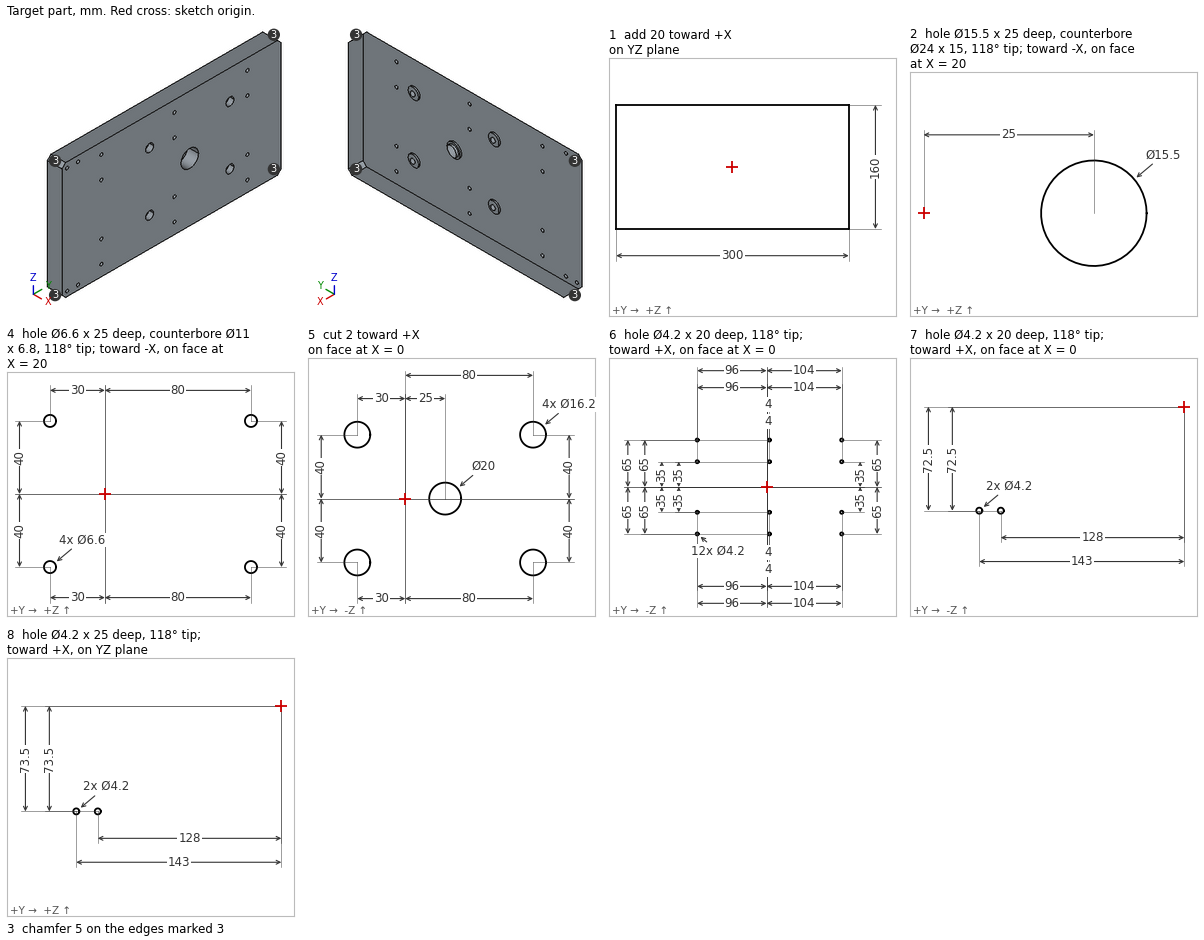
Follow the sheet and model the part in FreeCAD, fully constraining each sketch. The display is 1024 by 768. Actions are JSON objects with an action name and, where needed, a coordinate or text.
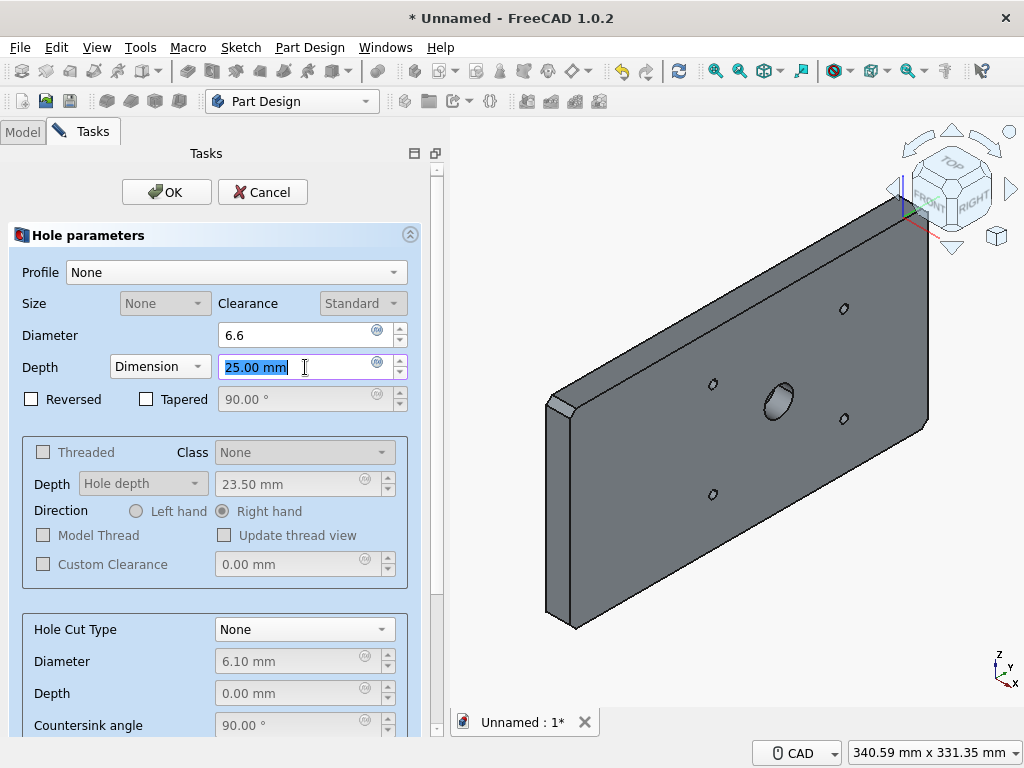
{"action": "type", "text": "25"}
{"action": "key", "text": "Tab"}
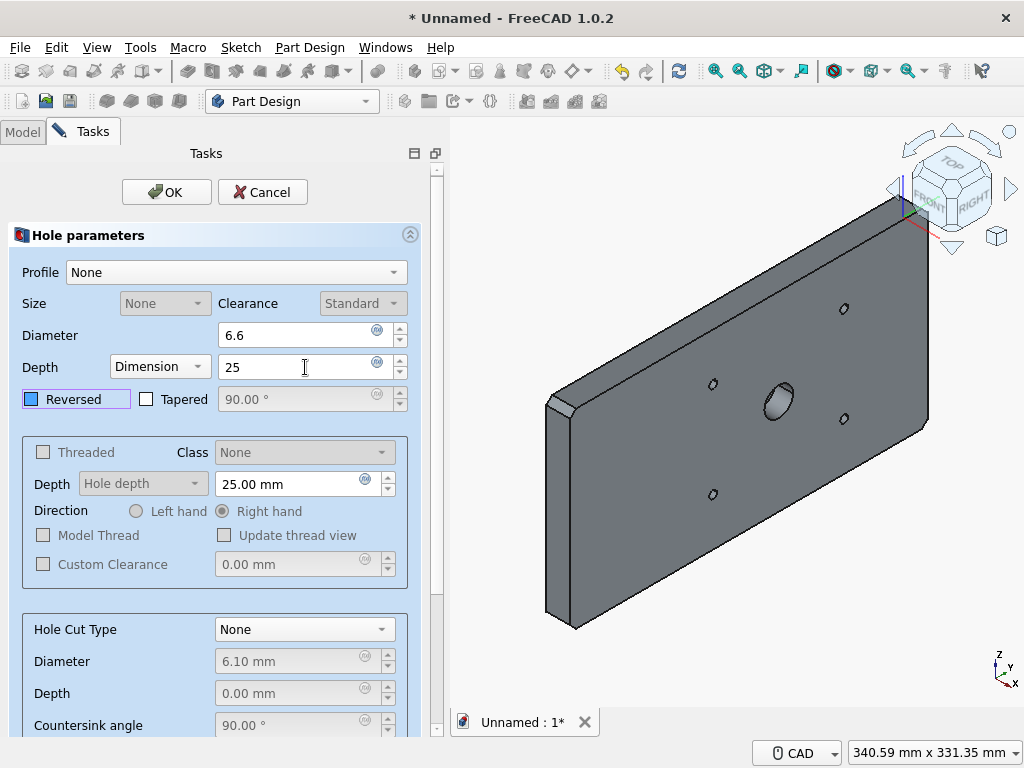
{"action": "left_click", "coordinate": [306, 630]}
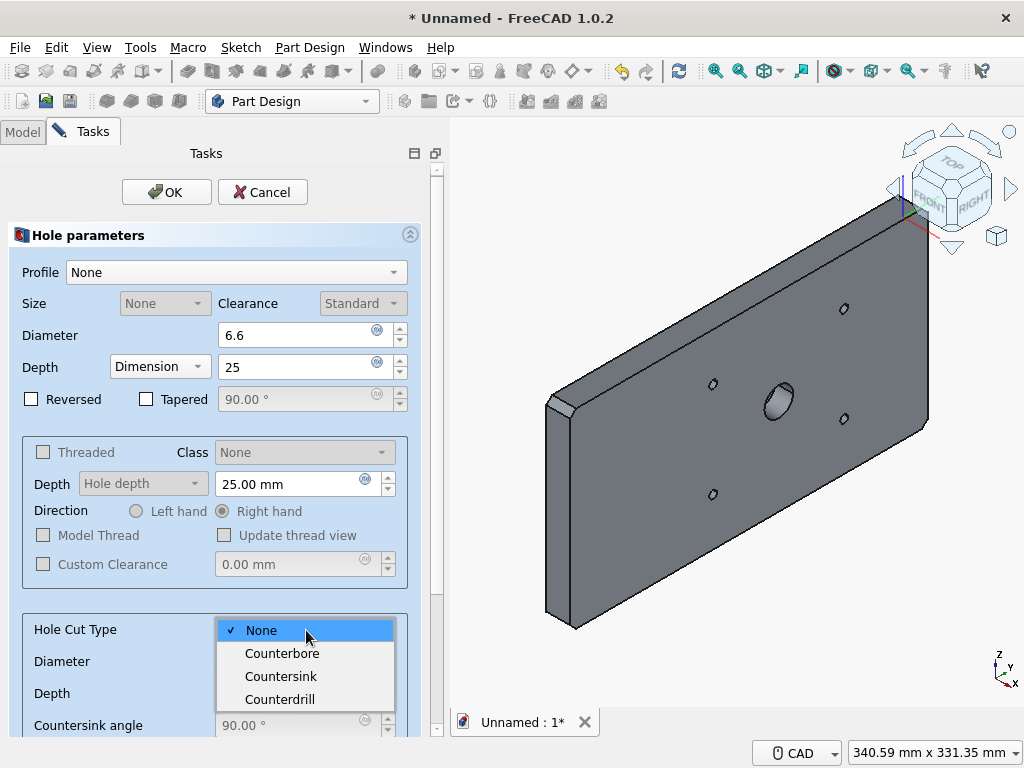
{"action": "left_click", "coordinate": [304, 654]}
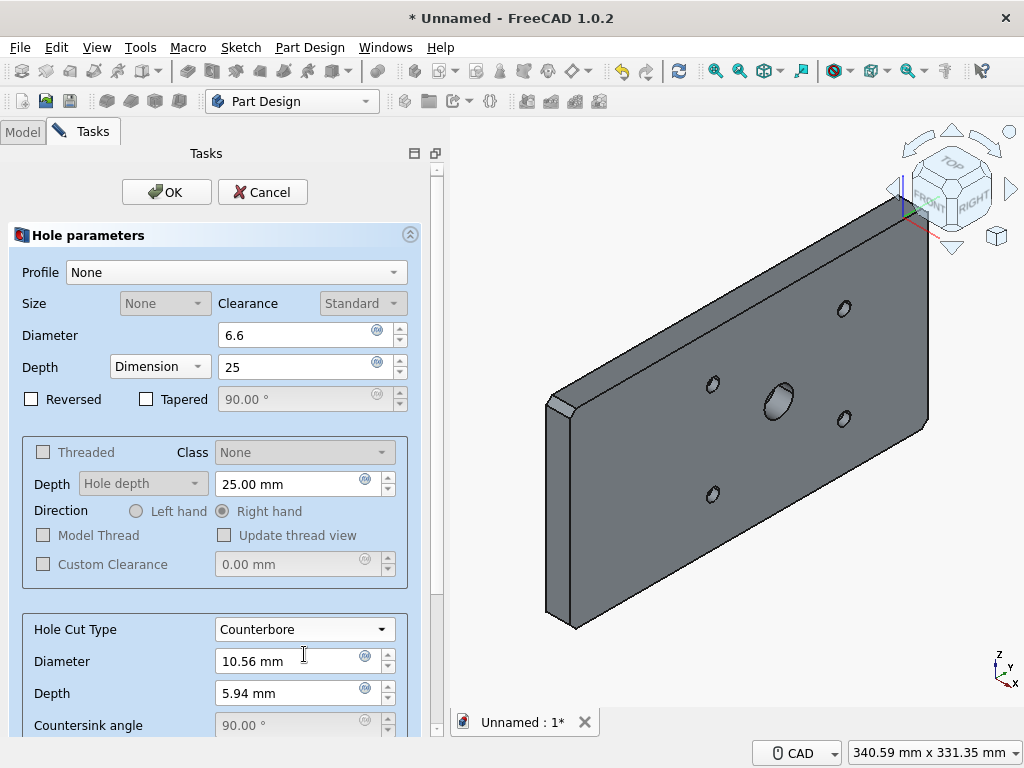
{"action": "triple_click", "coordinate": [298, 661]}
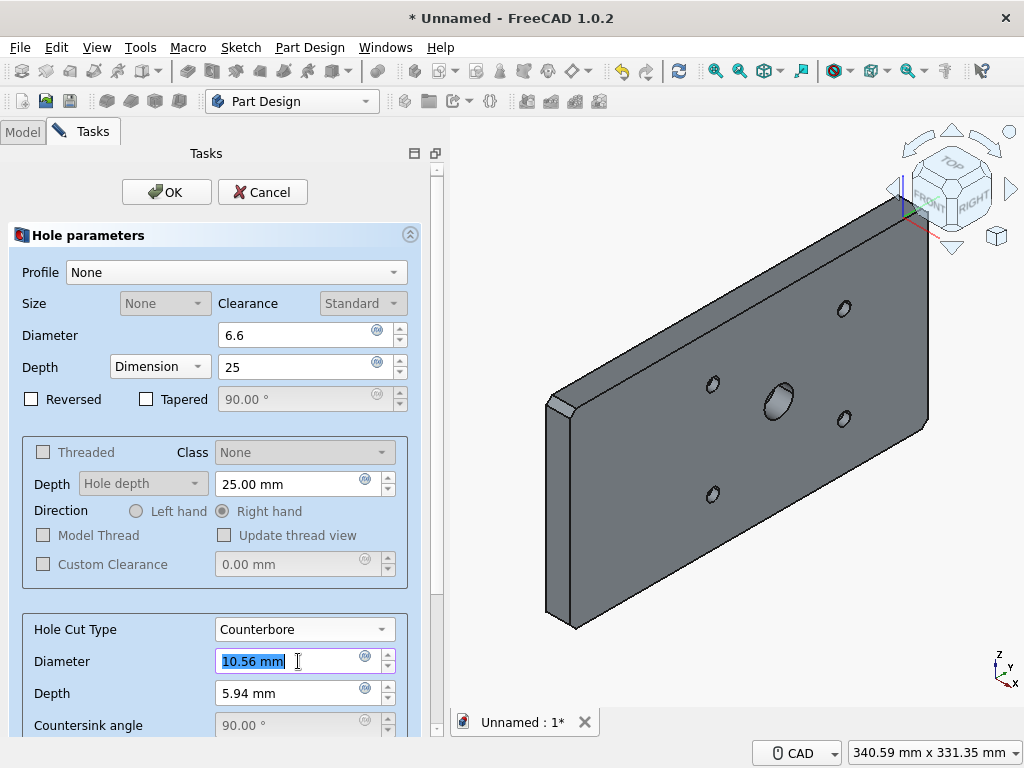
{"action": "type", "text": "11"}
{"action": "key", "text": "Tab"}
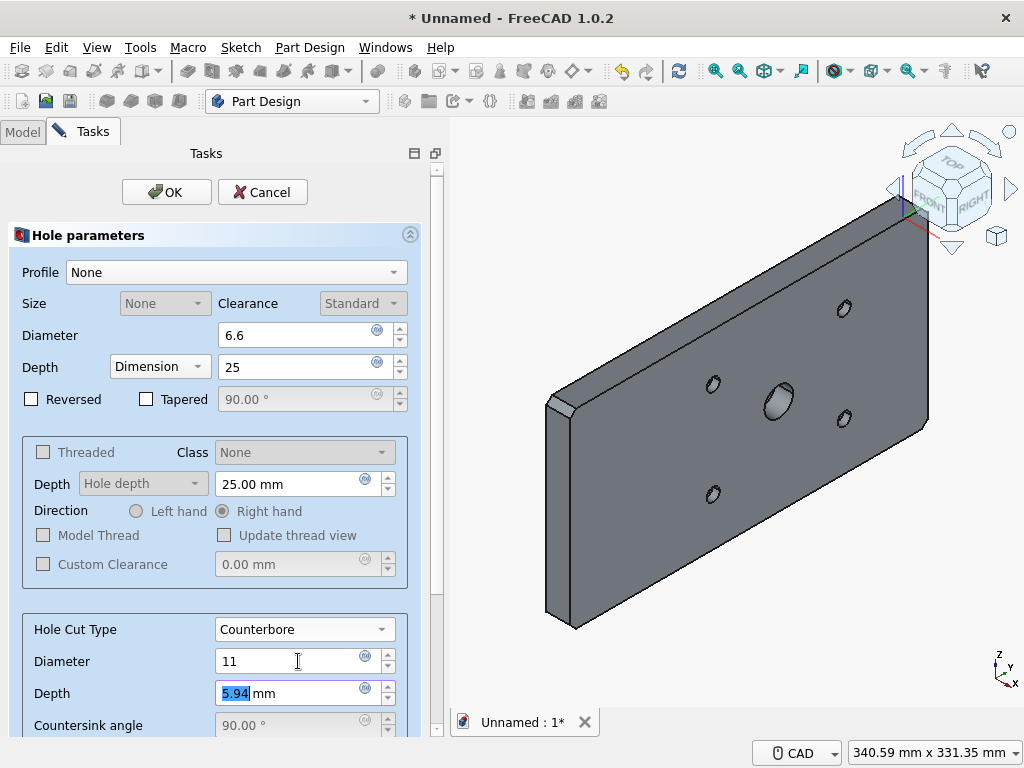
{"action": "type", "text": "6.8"}
{"action": "key", "text": "Tab"}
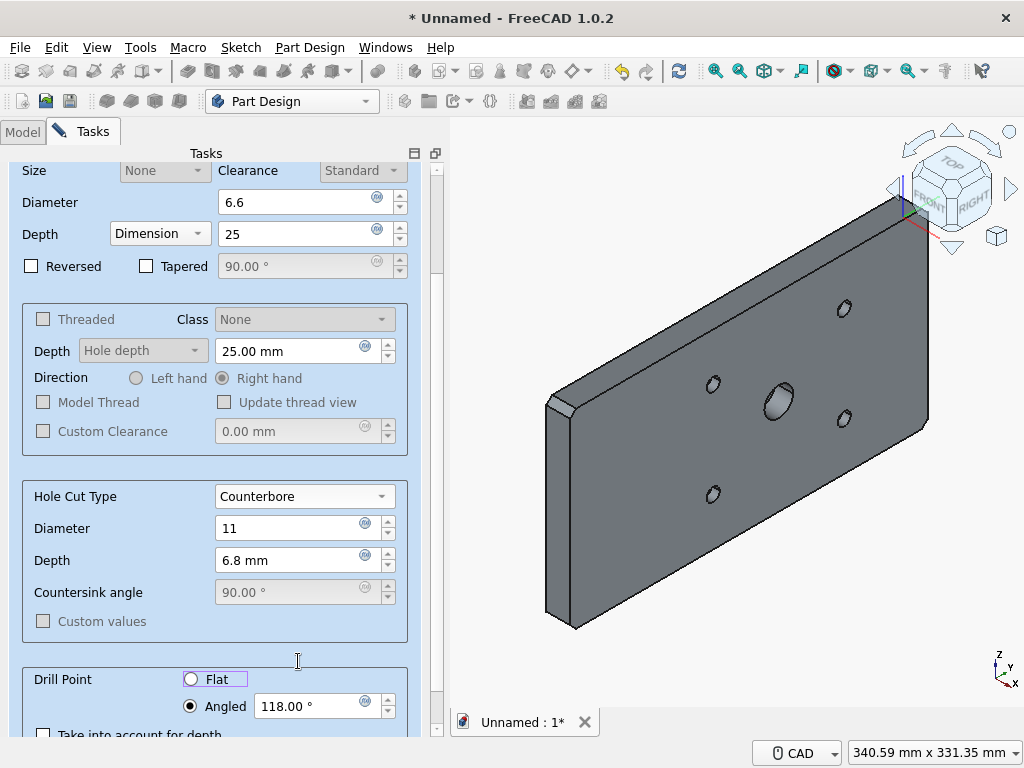
{"action": "scroll", "coordinate": [437, 450], "scroll_direction": "up", "scroll_amount": 3}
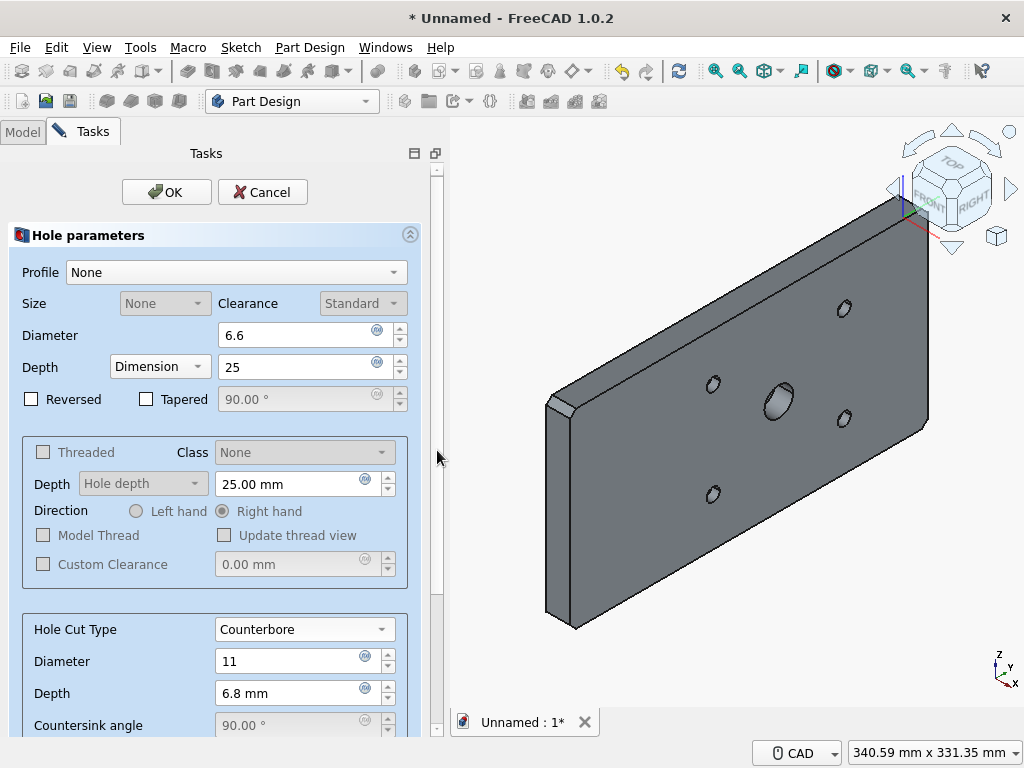
{"action": "left_click", "coordinate": [167, 192]}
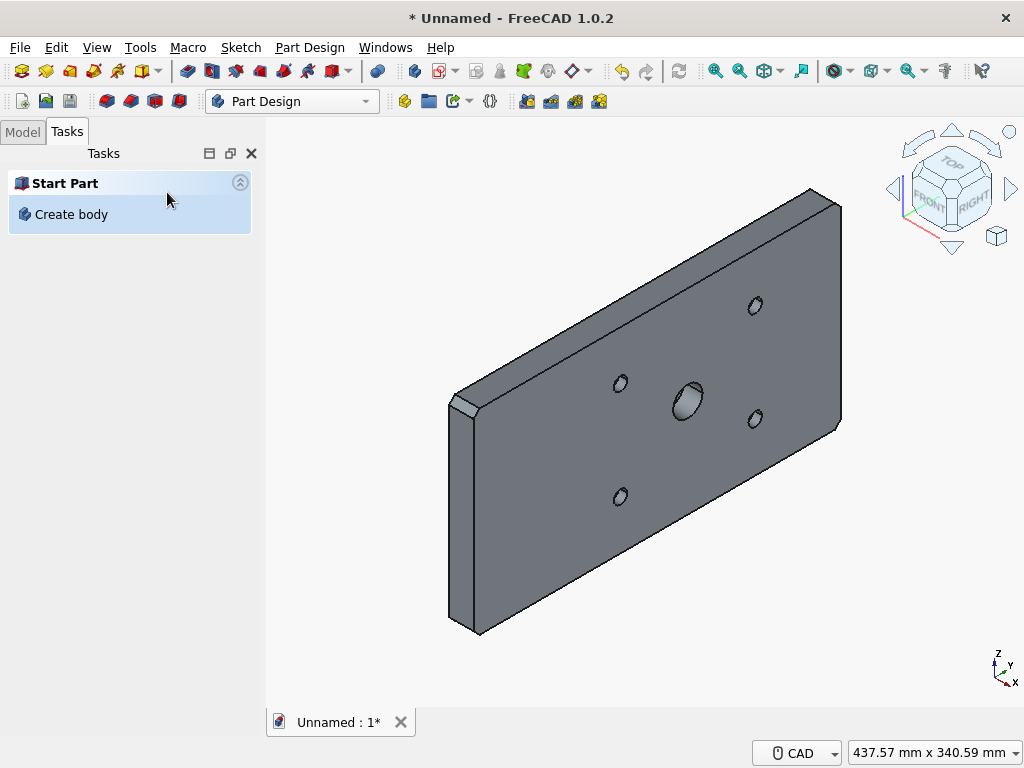
{"action": "key", "text": "6"}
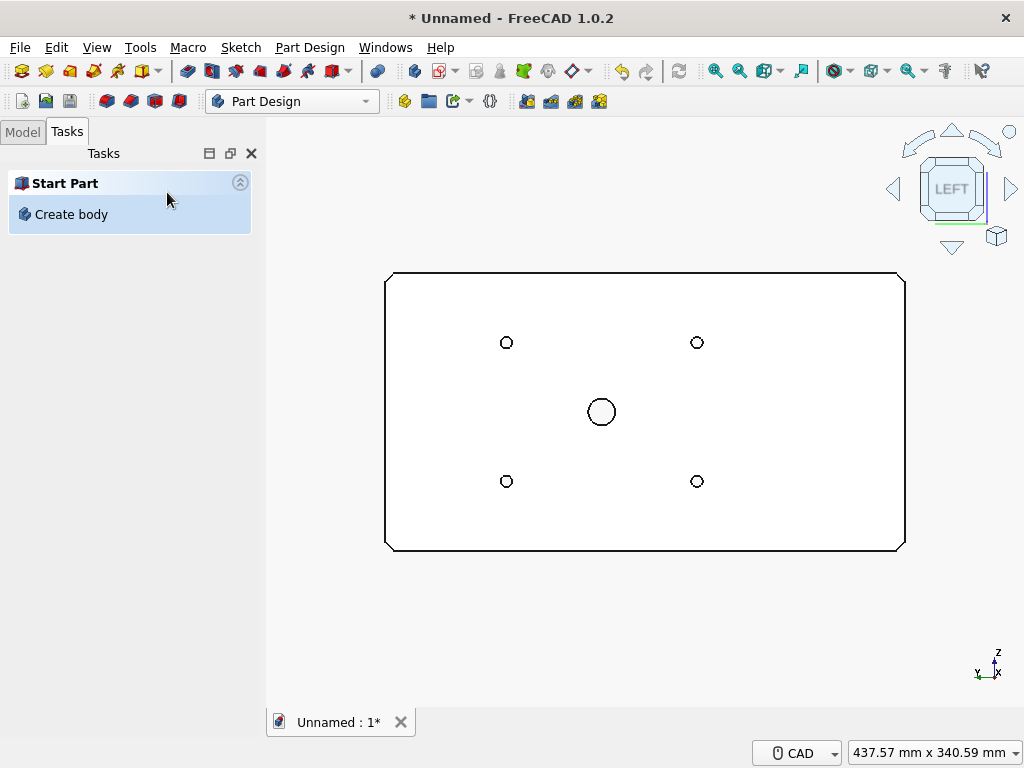
{"action": "left_click", "coordinate": [793, 411]}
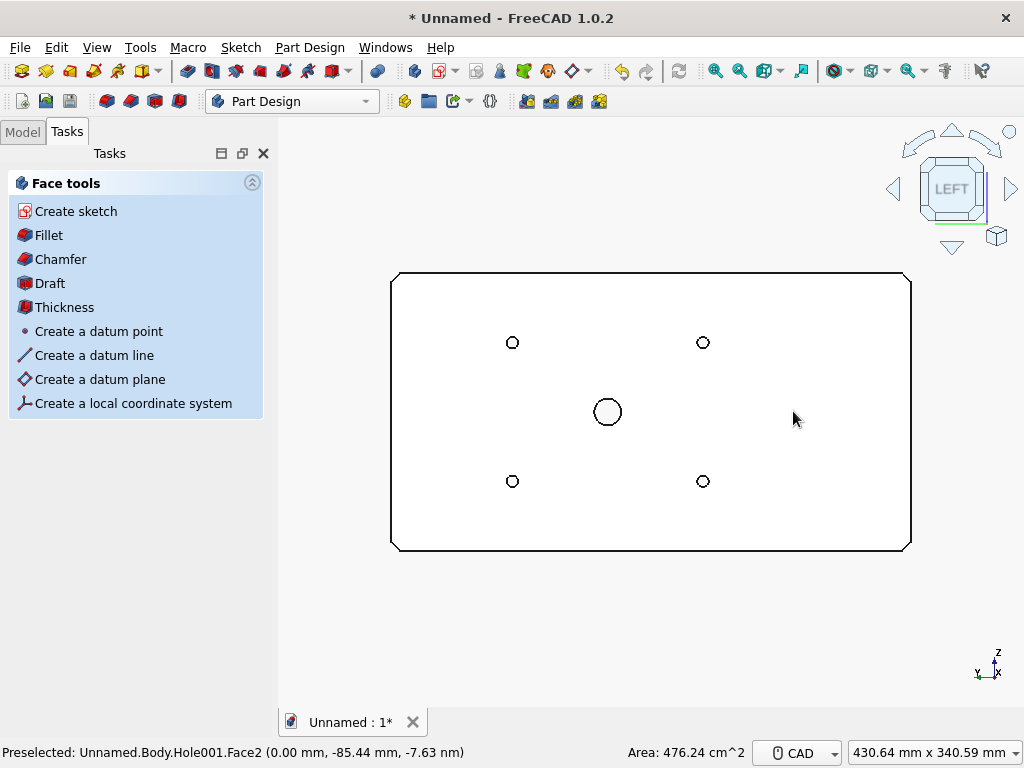
{"action": "left_click", "coordinate": [440, 72]}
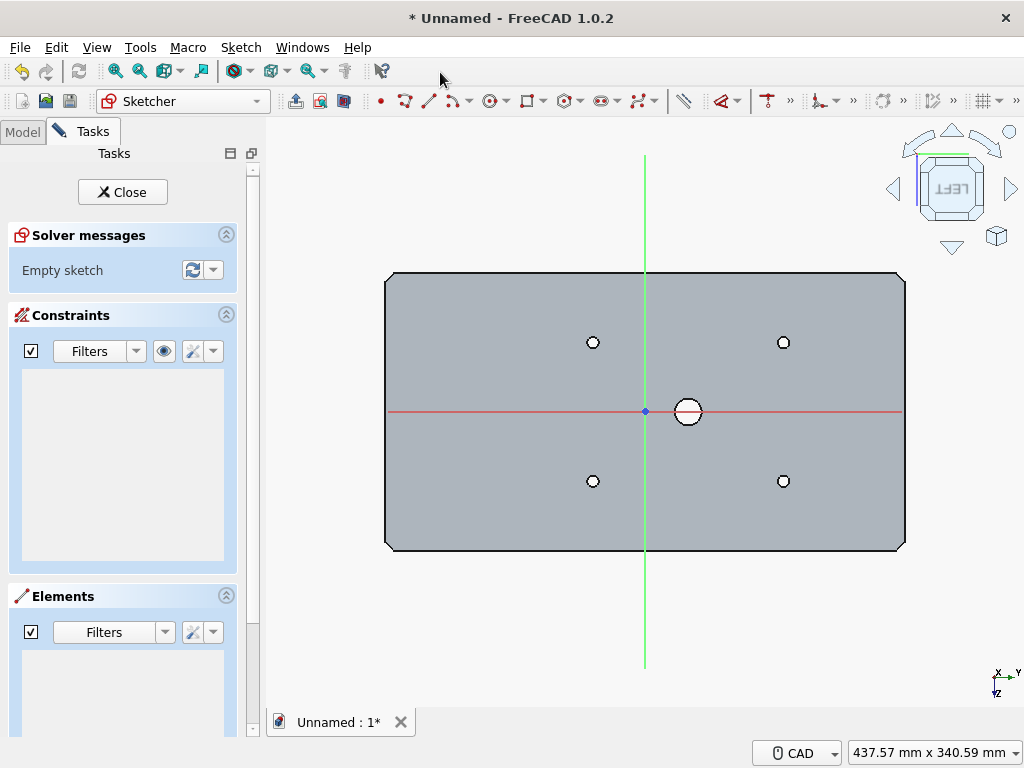
{"action": "scroll", "coordinate": [824, 412], "scroll_direction": "up", "scroll_amount": 3}